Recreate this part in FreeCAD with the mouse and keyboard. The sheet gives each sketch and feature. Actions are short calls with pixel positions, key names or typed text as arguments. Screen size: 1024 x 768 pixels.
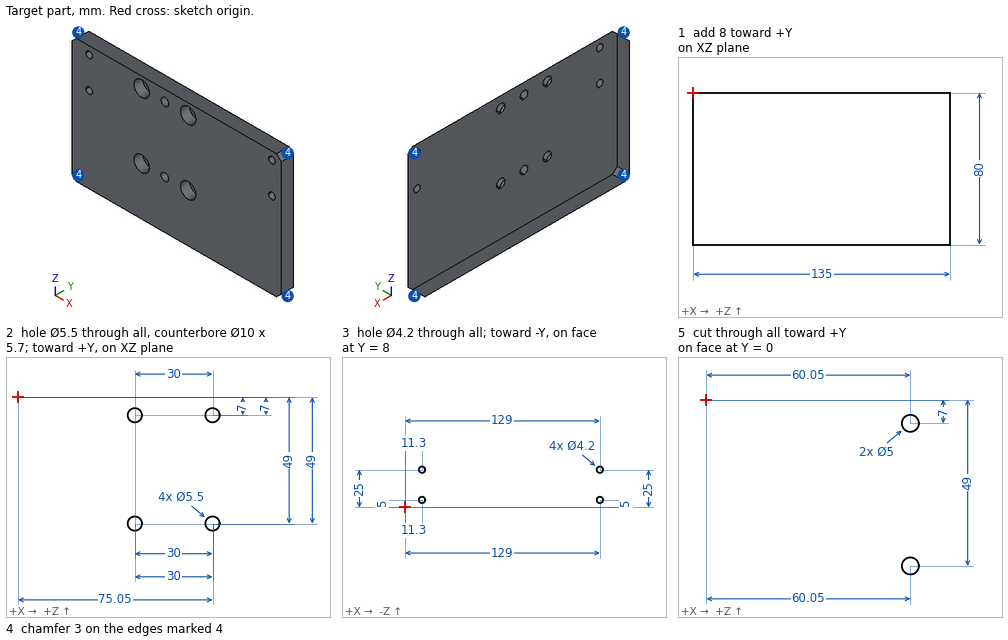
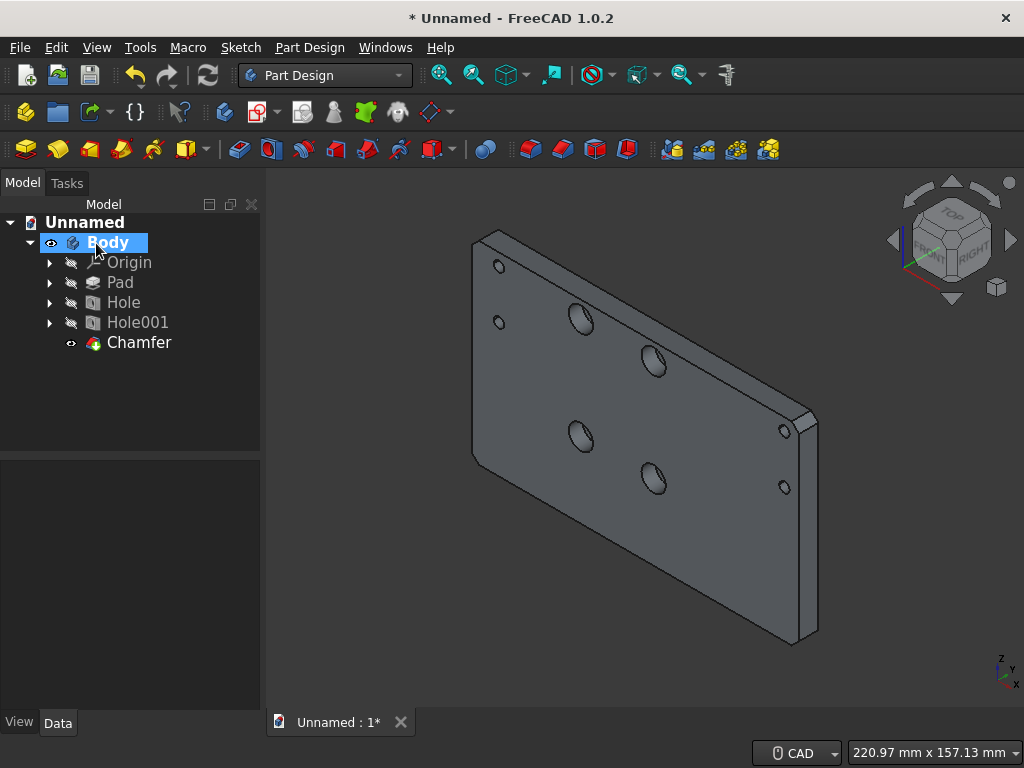
click(729, 528)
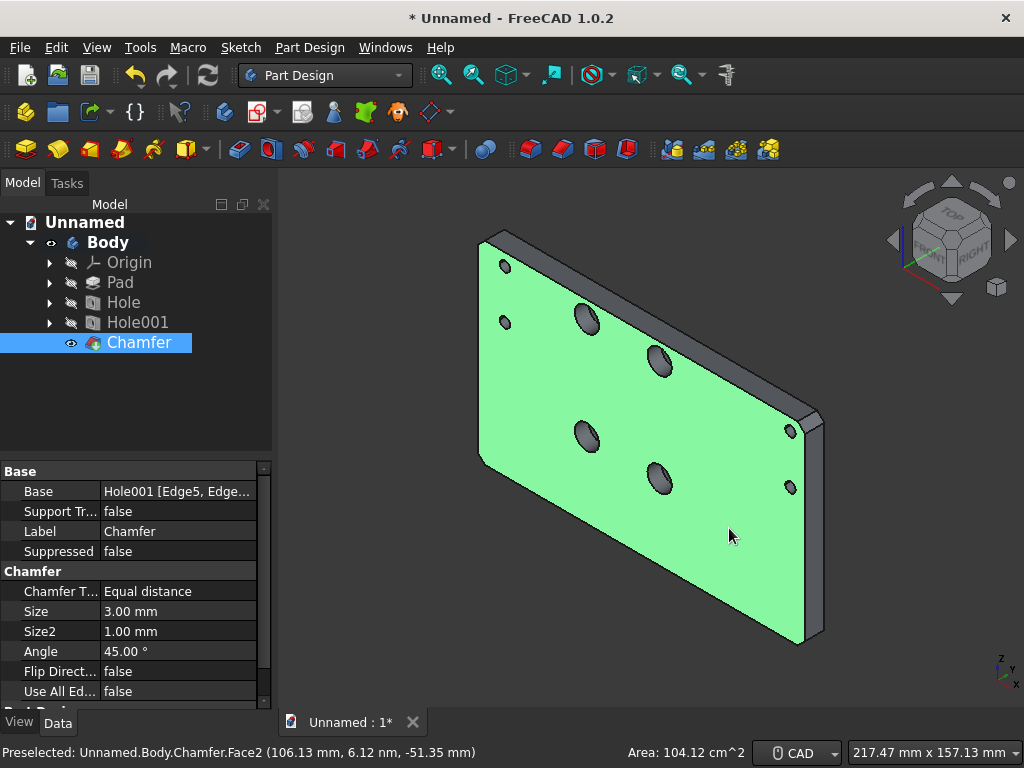
click(258, 112)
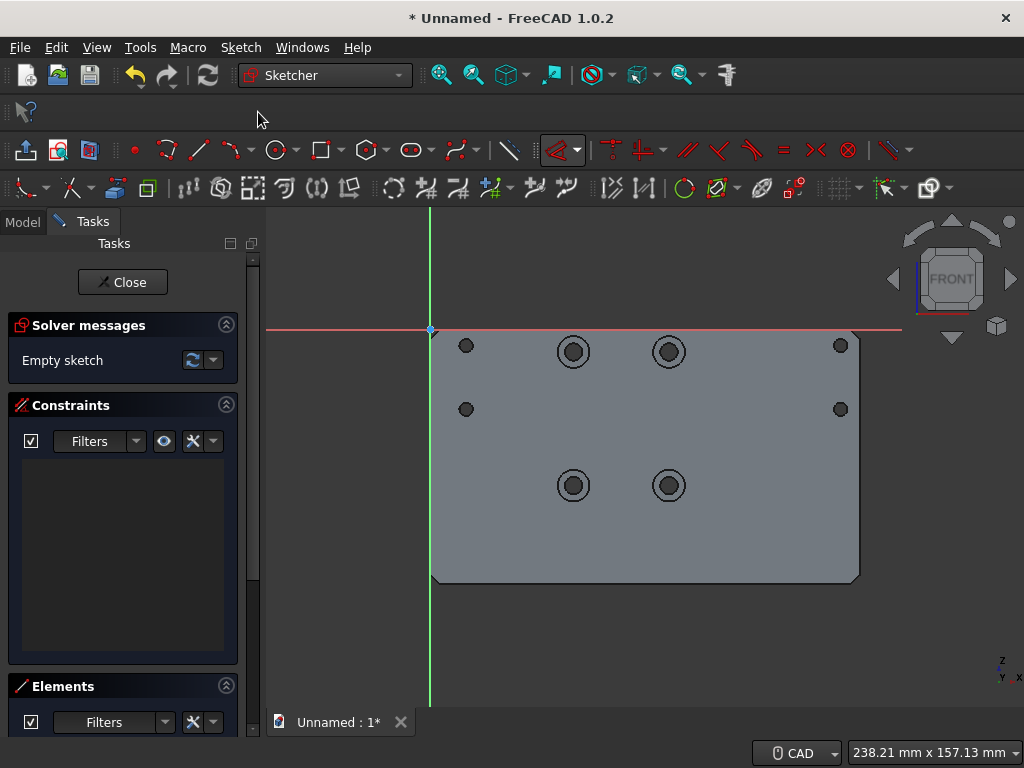
scroll(473, 356, up, 3)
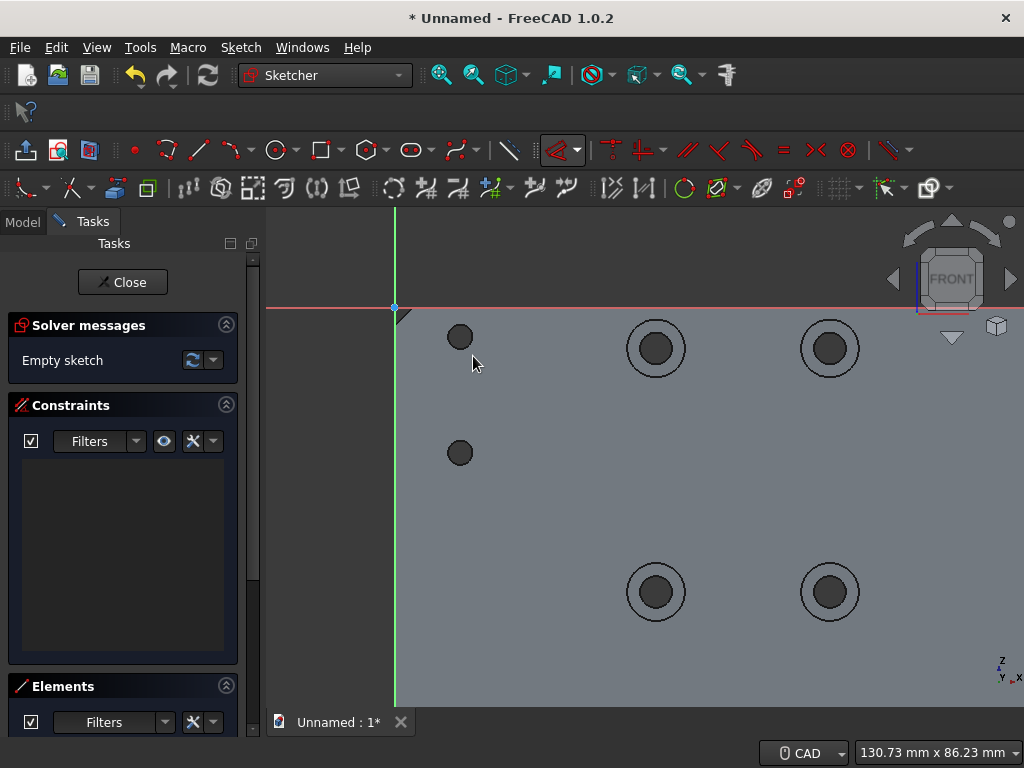
key(g)
key(c)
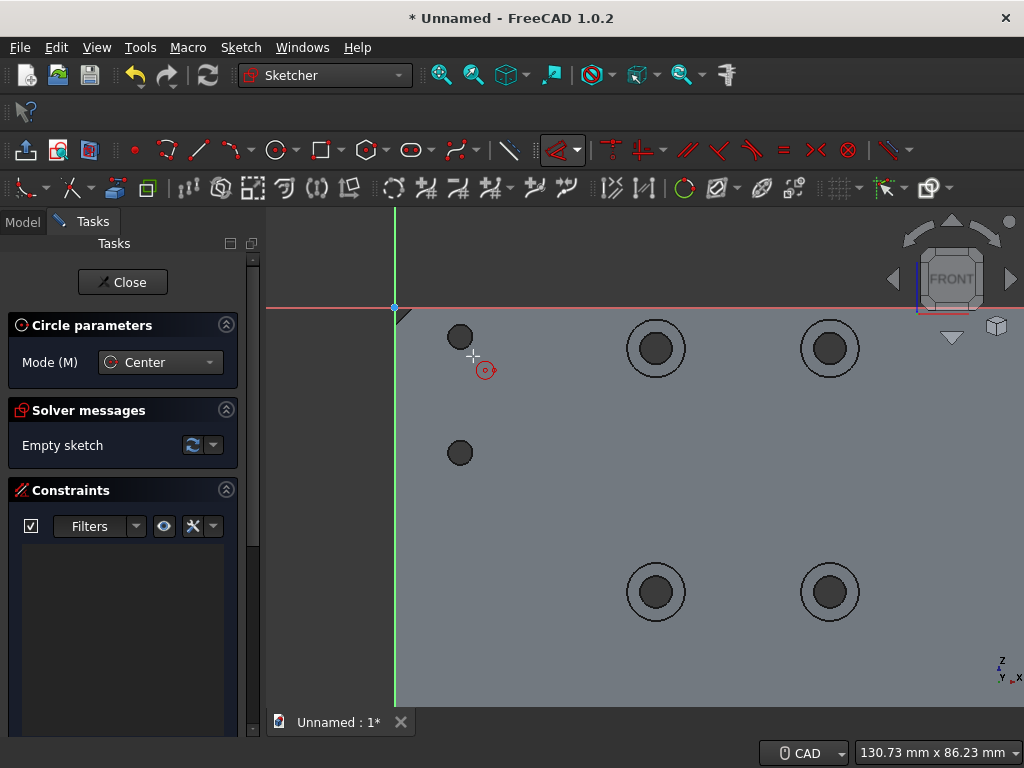
scroll(743, 348, up, 3)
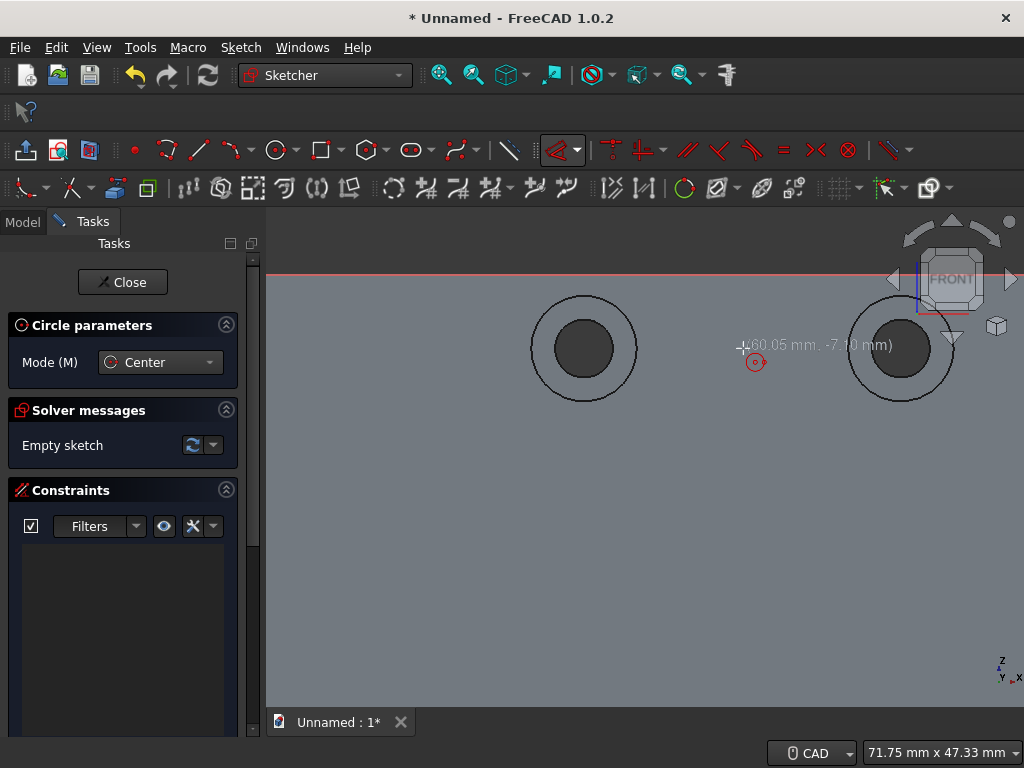
click(742, 349)
move(761, 330)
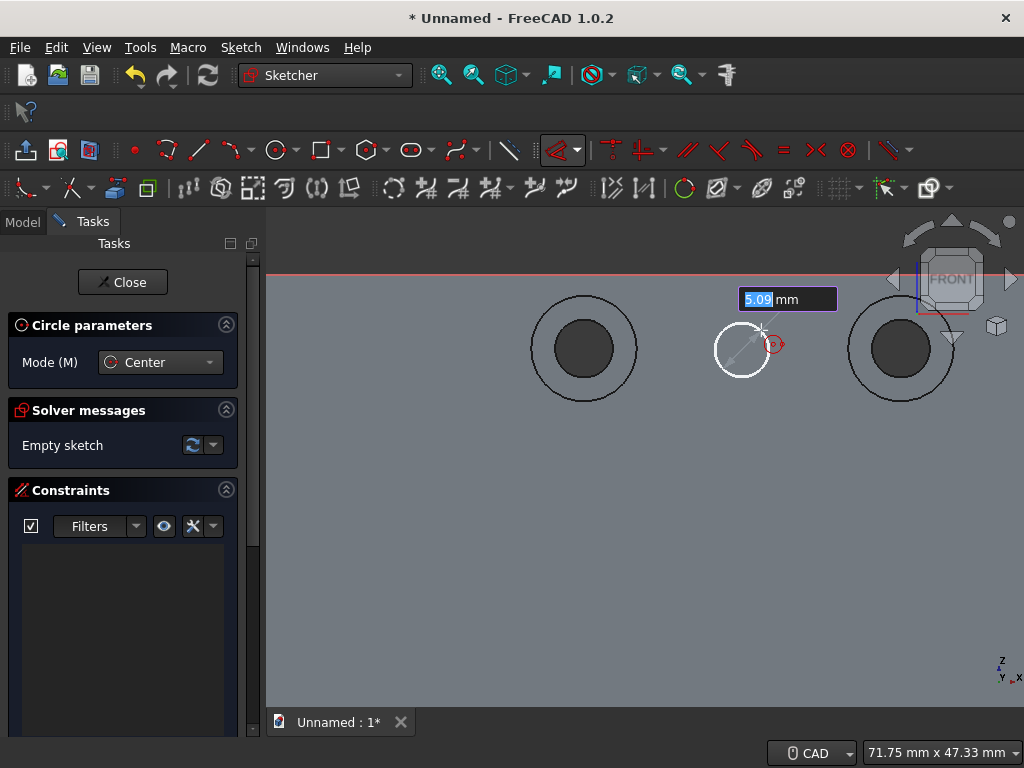
text(5)
key(Return)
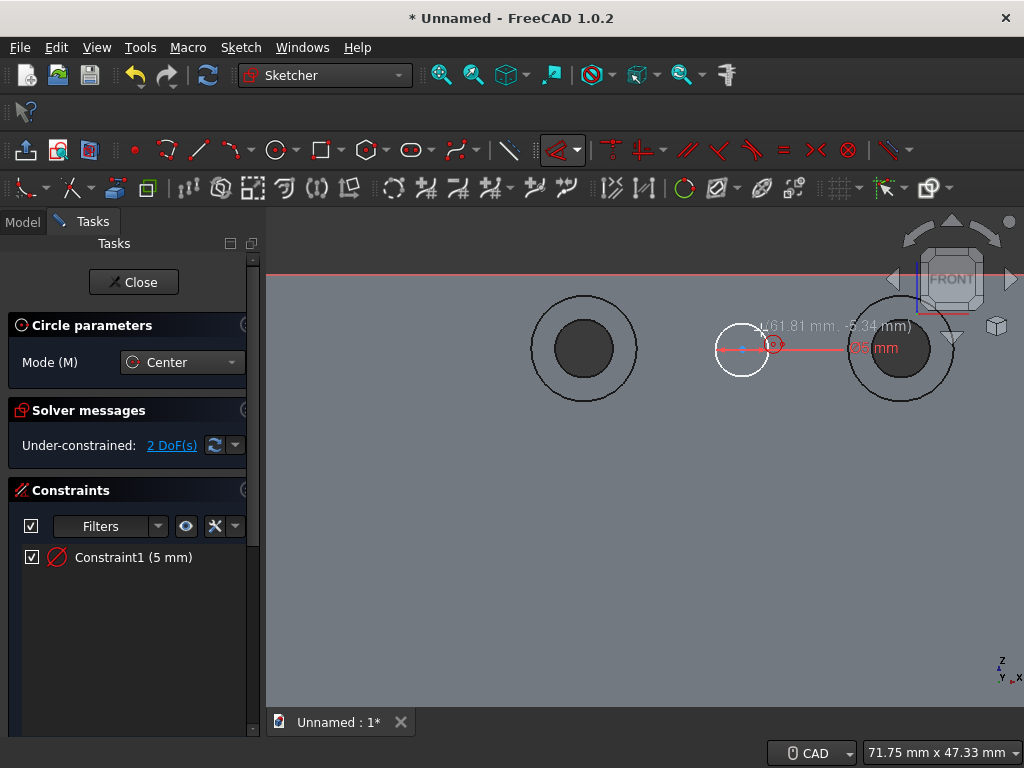
scroll(744, 348, down, 3)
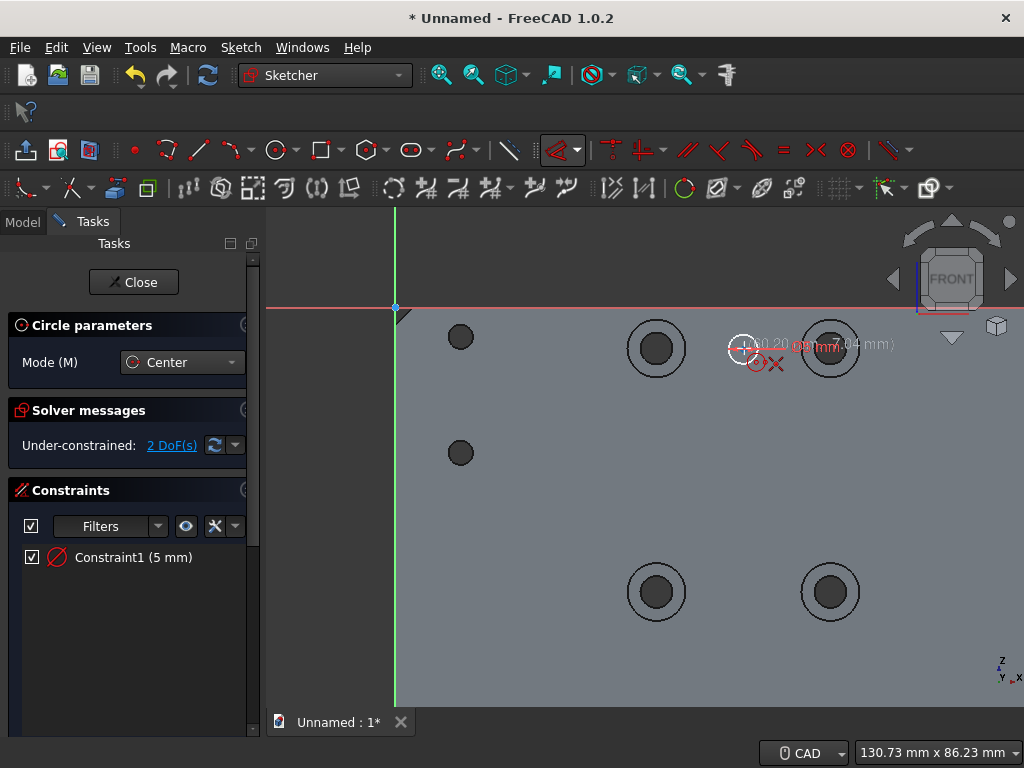
scroll(743, 592, up, 3)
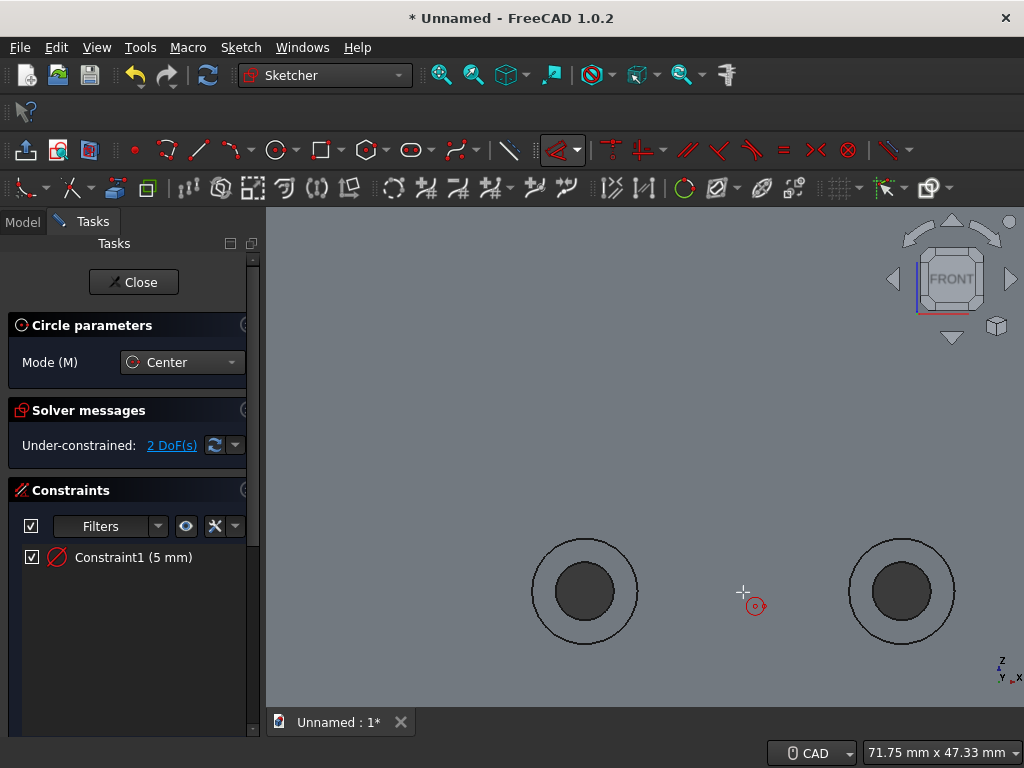
click(743, 591)
move(762, 573)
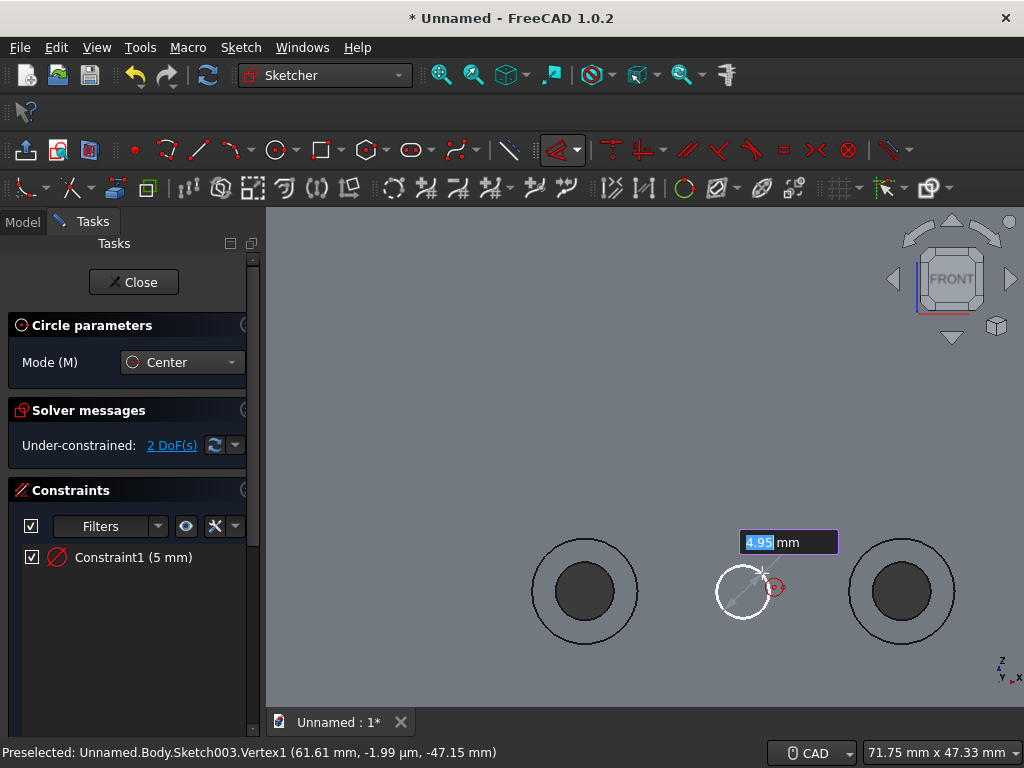
text(5)
key(Return)
key(Escape)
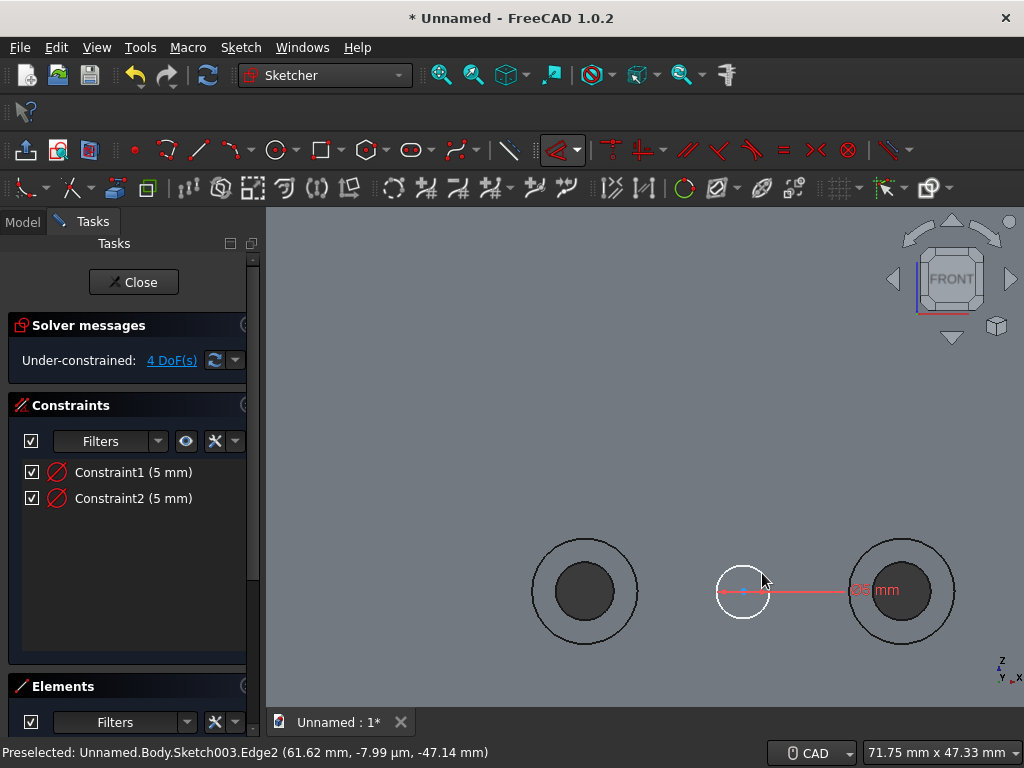
scroll(743, 592, down, 3)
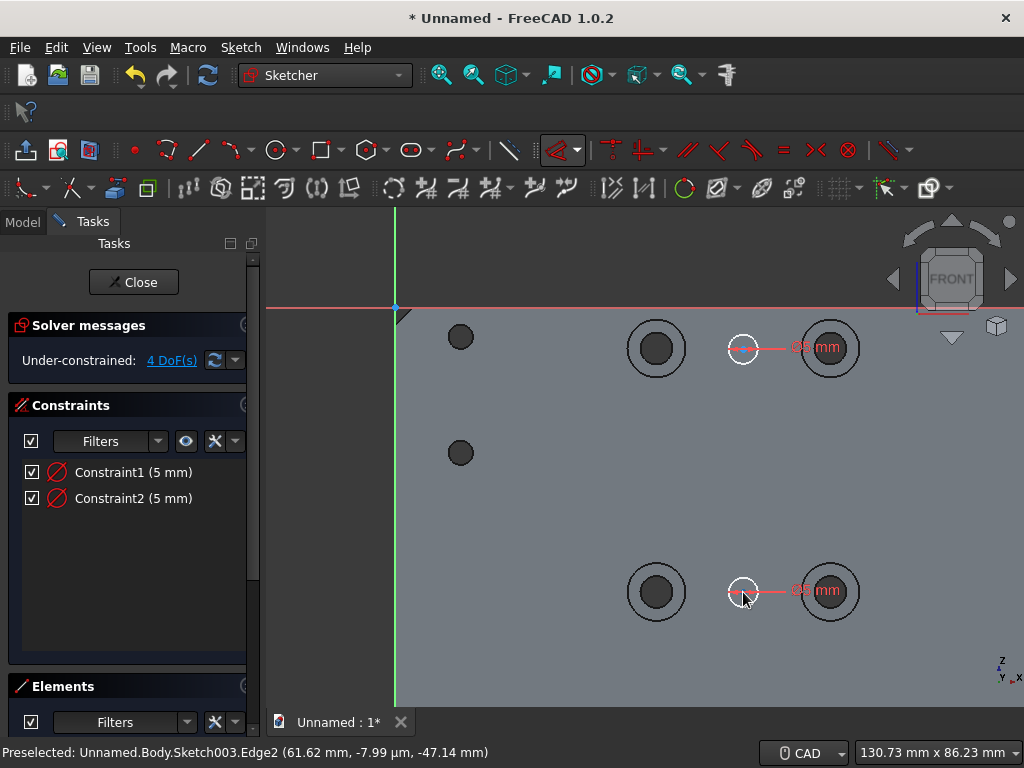
click(743, 349)